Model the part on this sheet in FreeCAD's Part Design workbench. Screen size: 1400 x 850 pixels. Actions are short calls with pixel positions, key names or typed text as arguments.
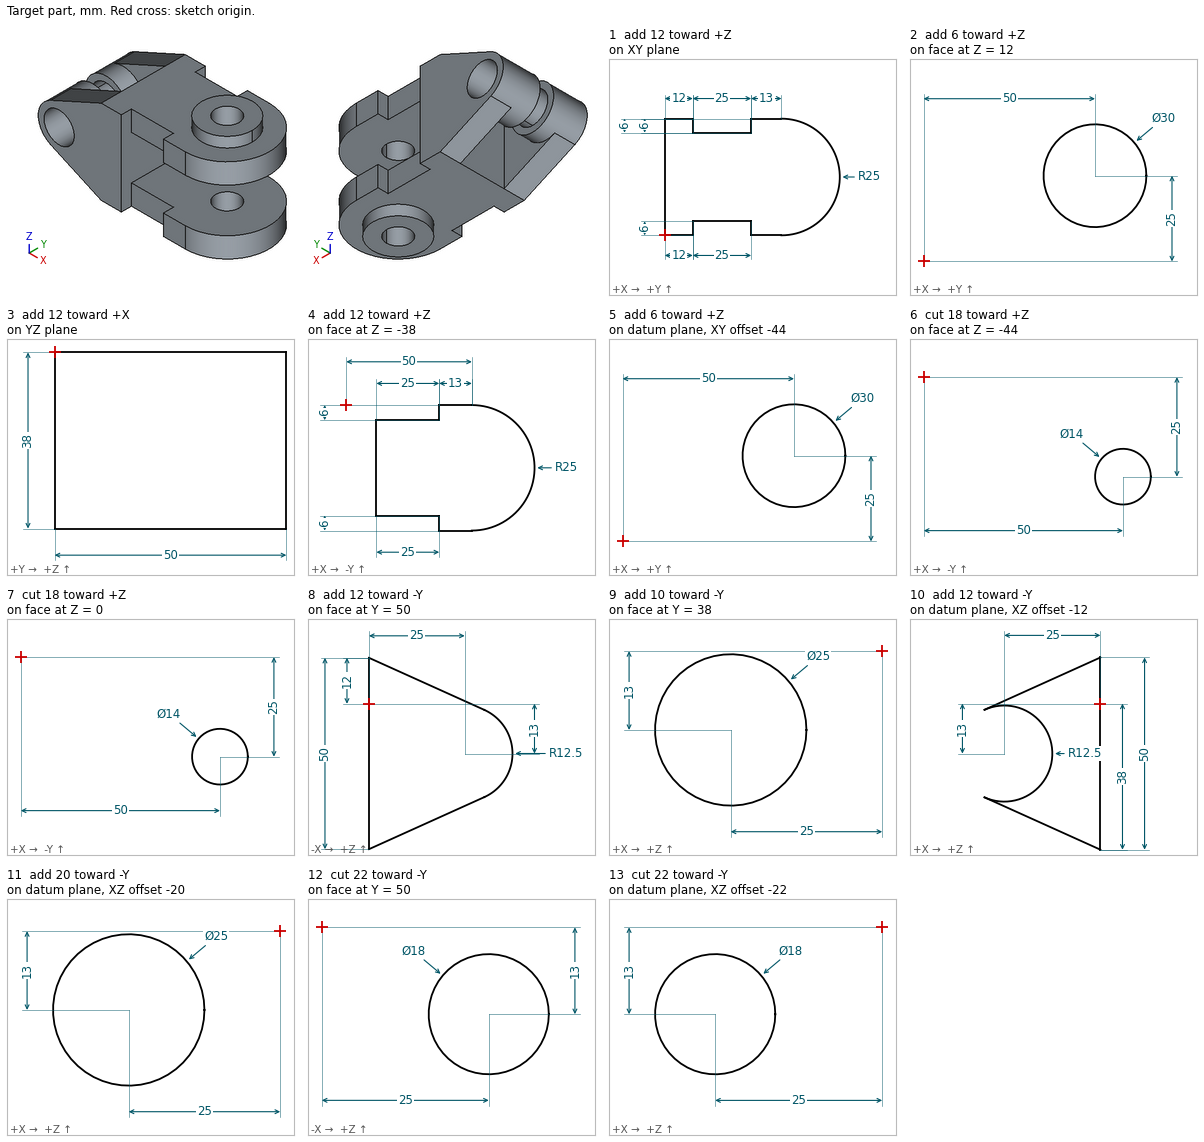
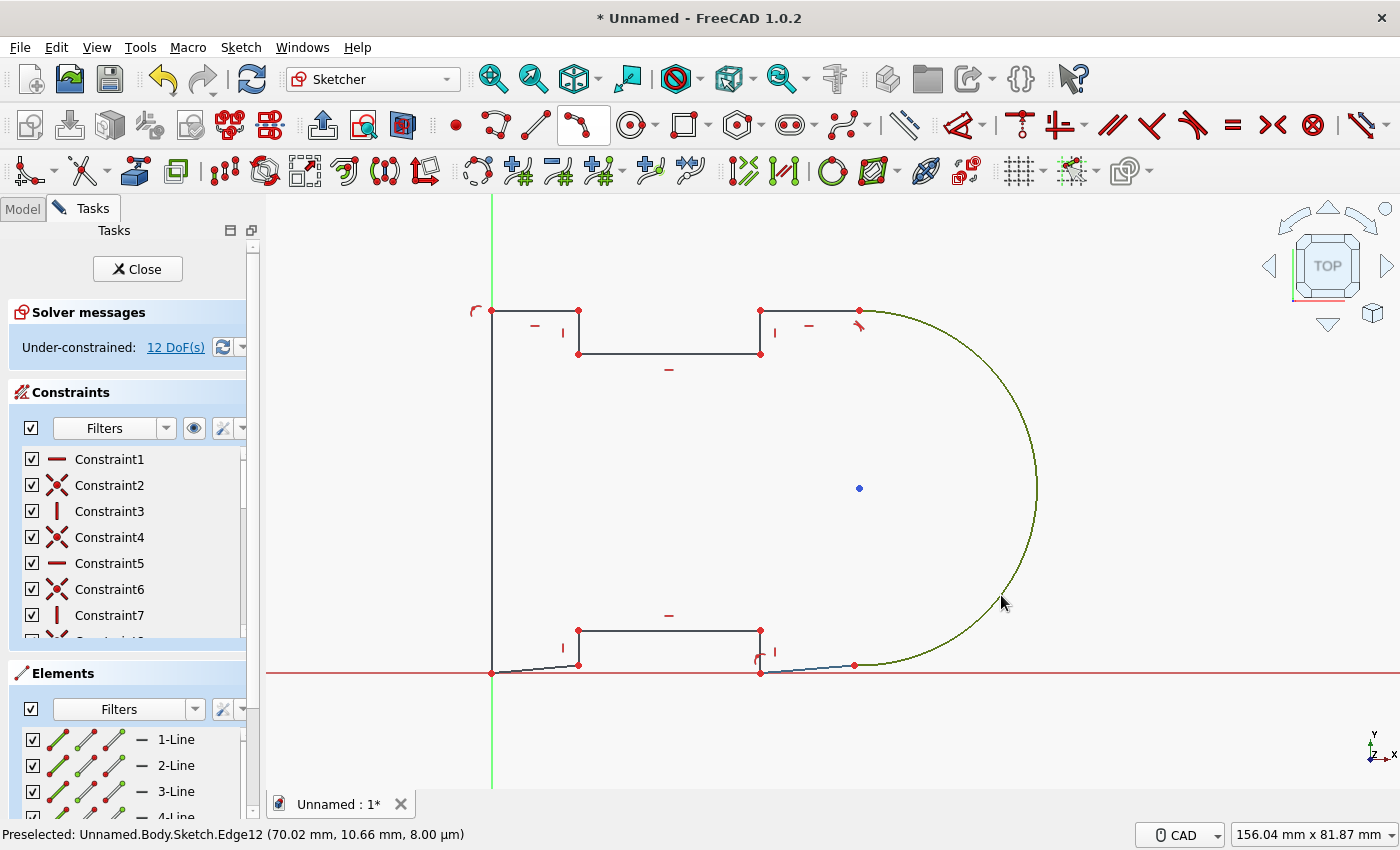
click(1194, 126)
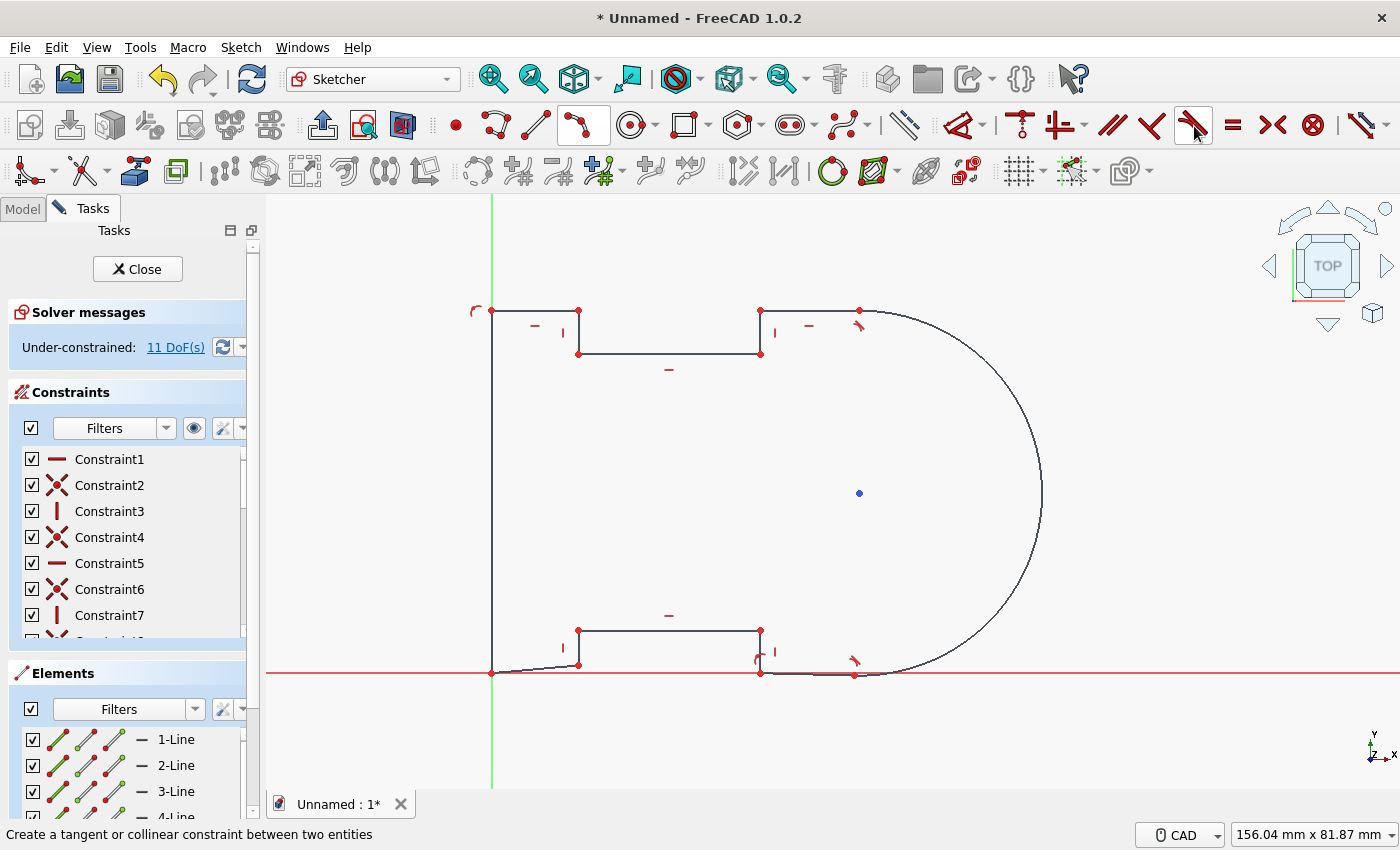
click(518, 671)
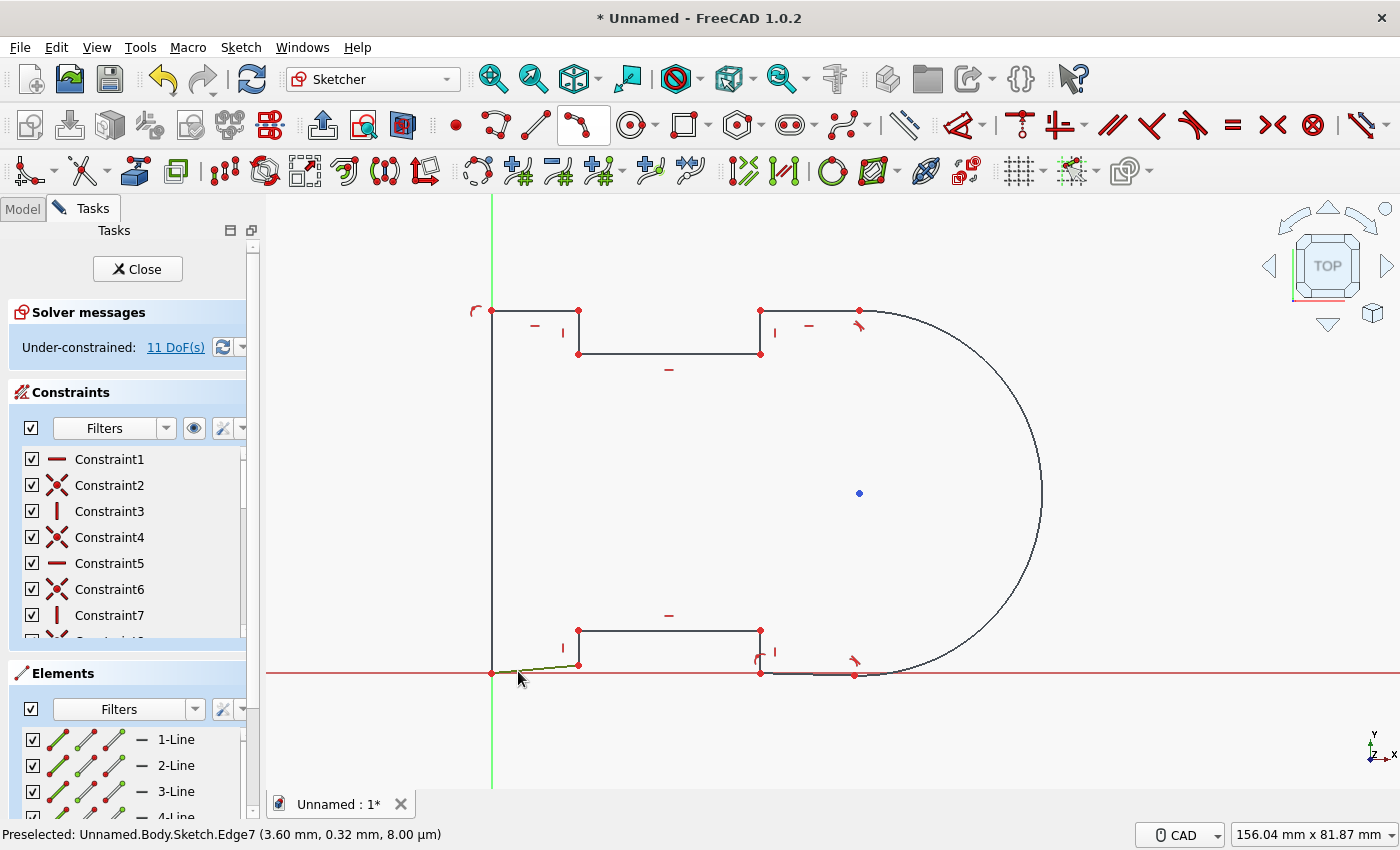
key(h)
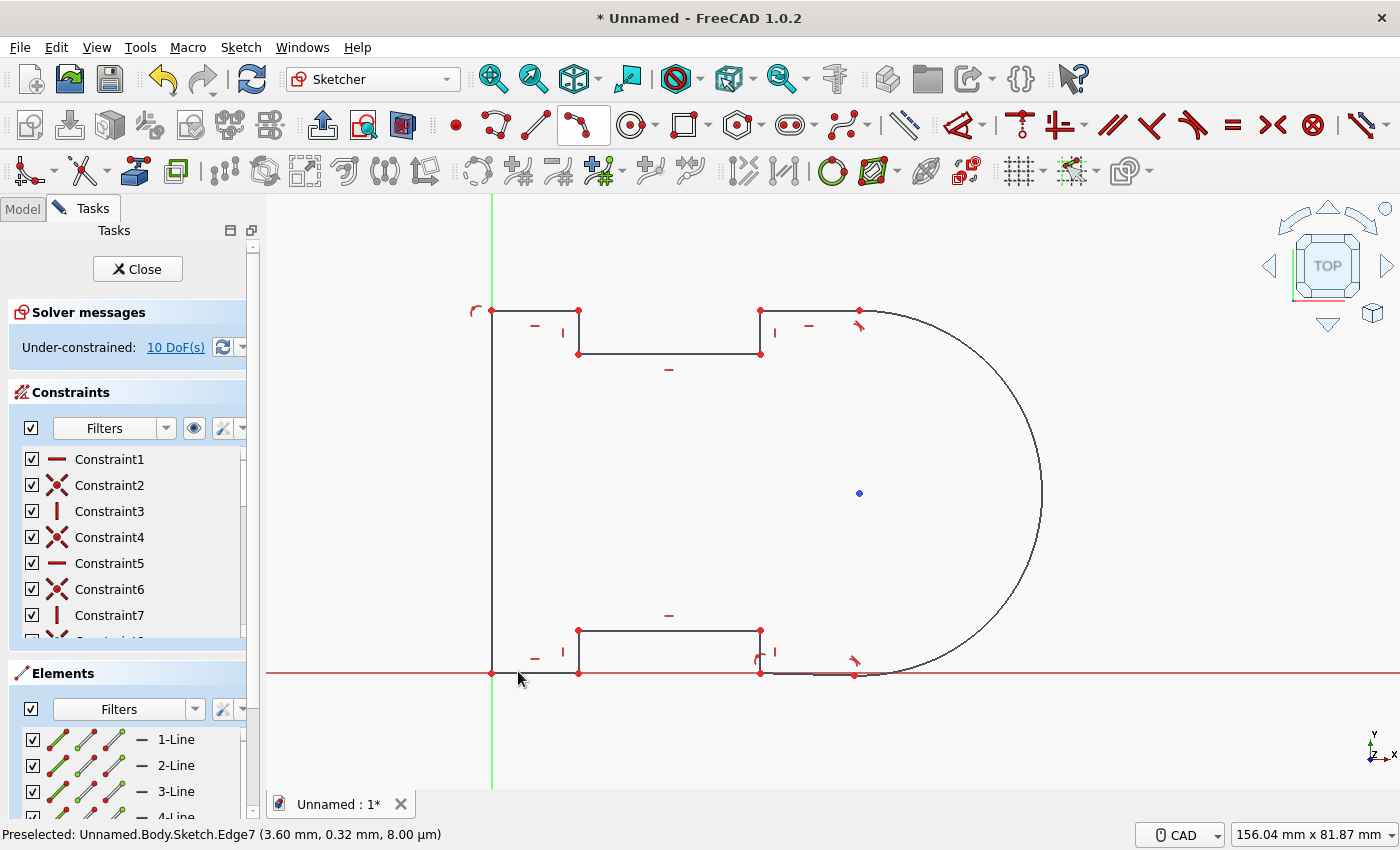
click(789, 674)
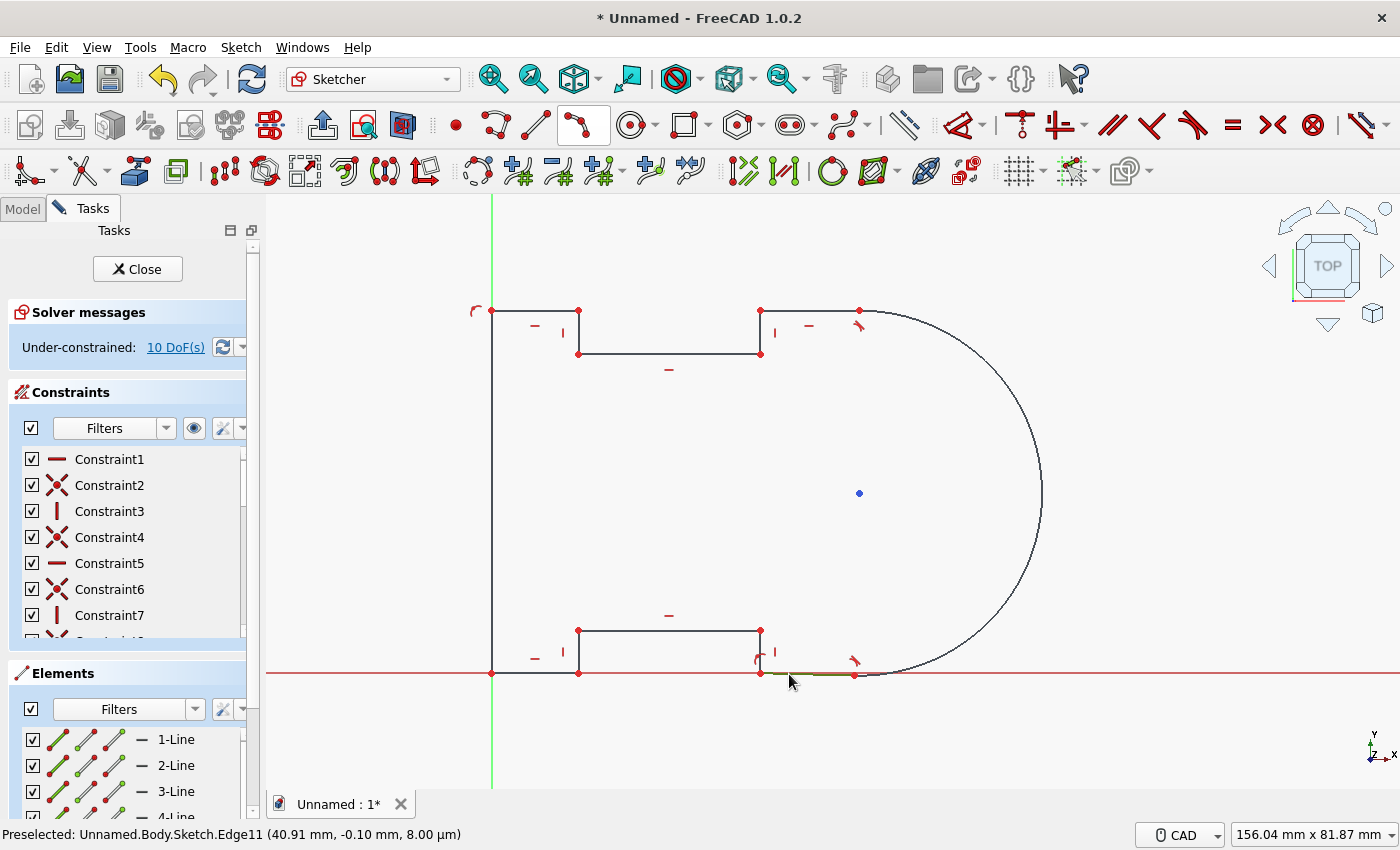
click(1086, 126)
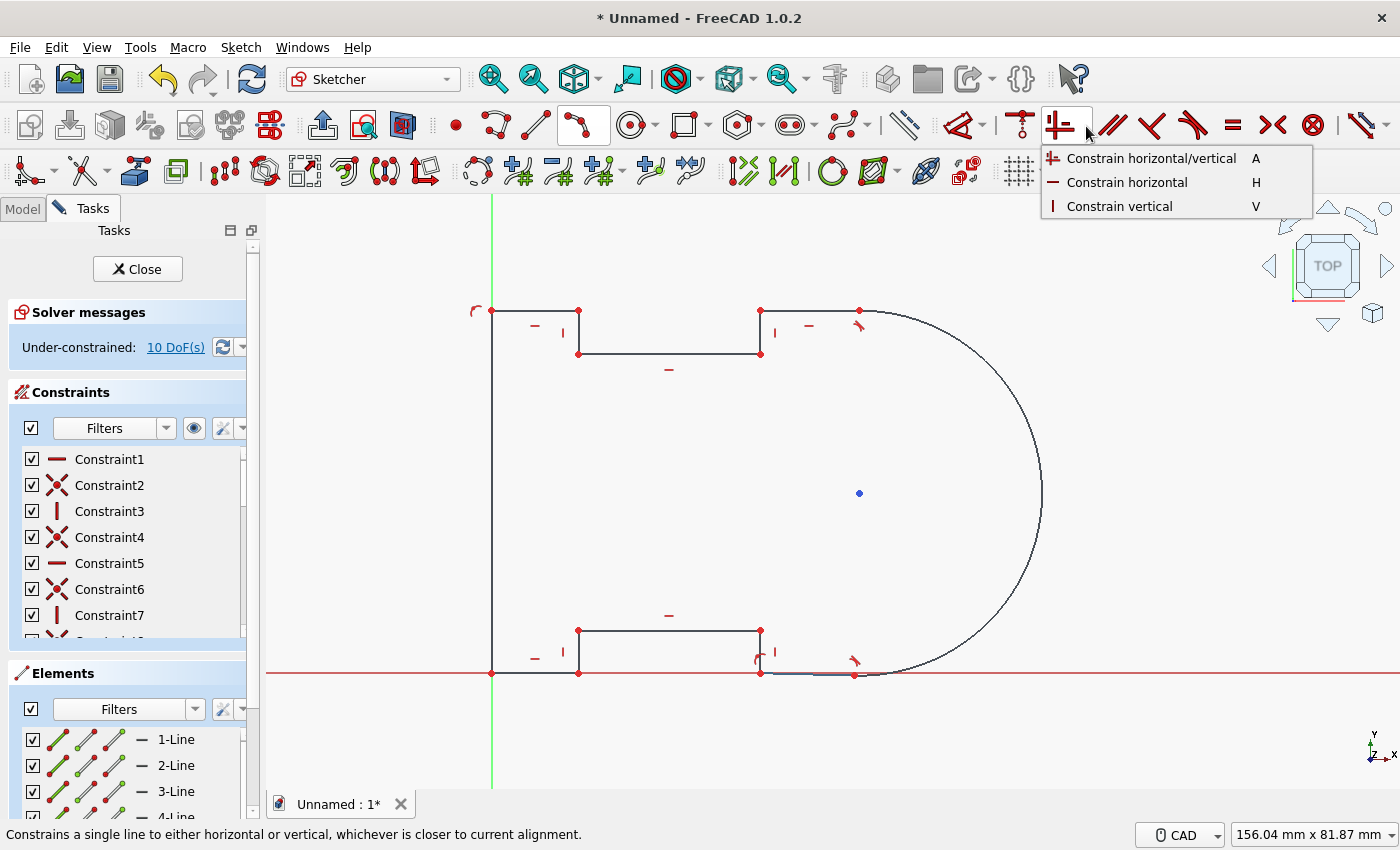
click(1177, 182)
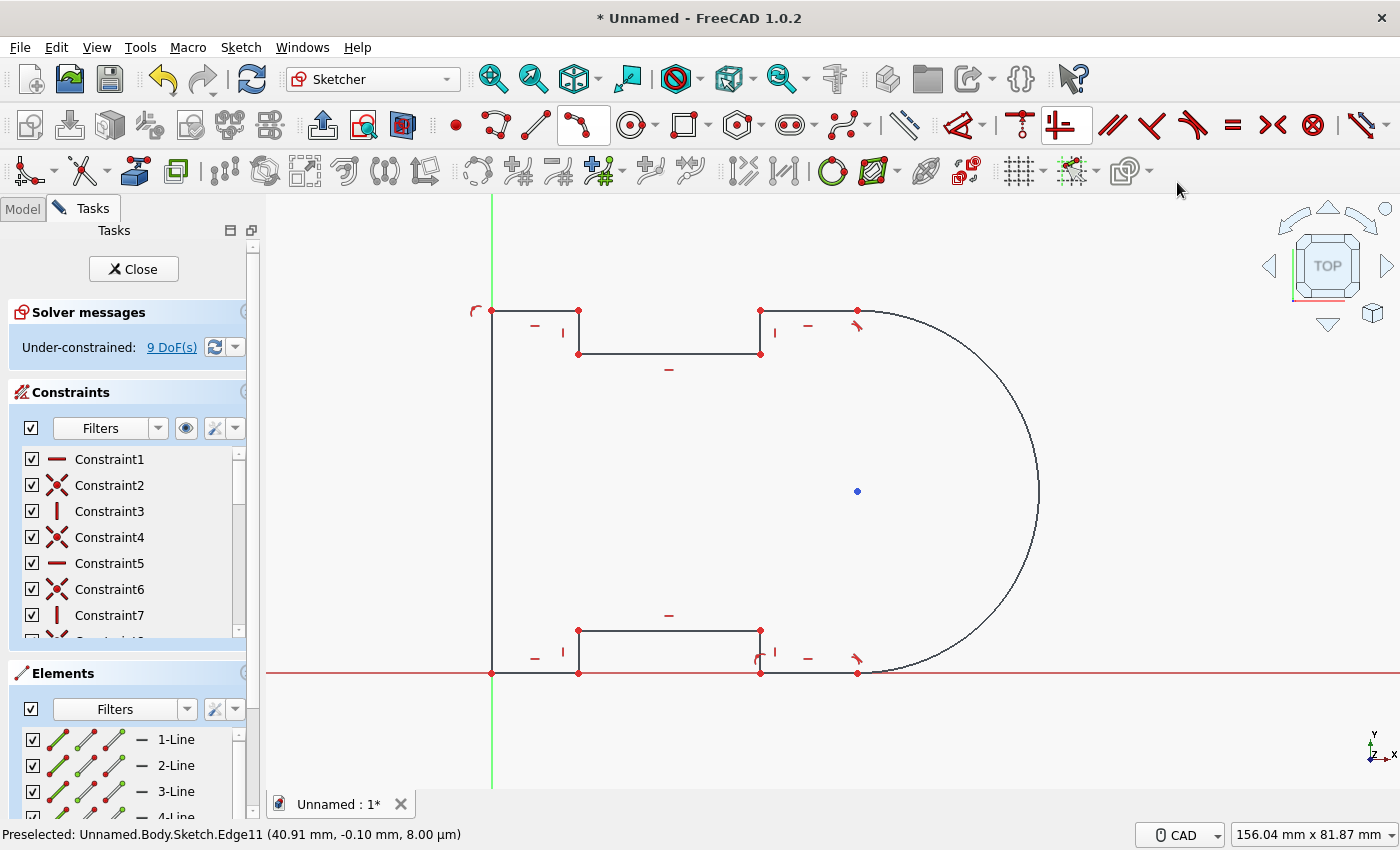
click(958, 126)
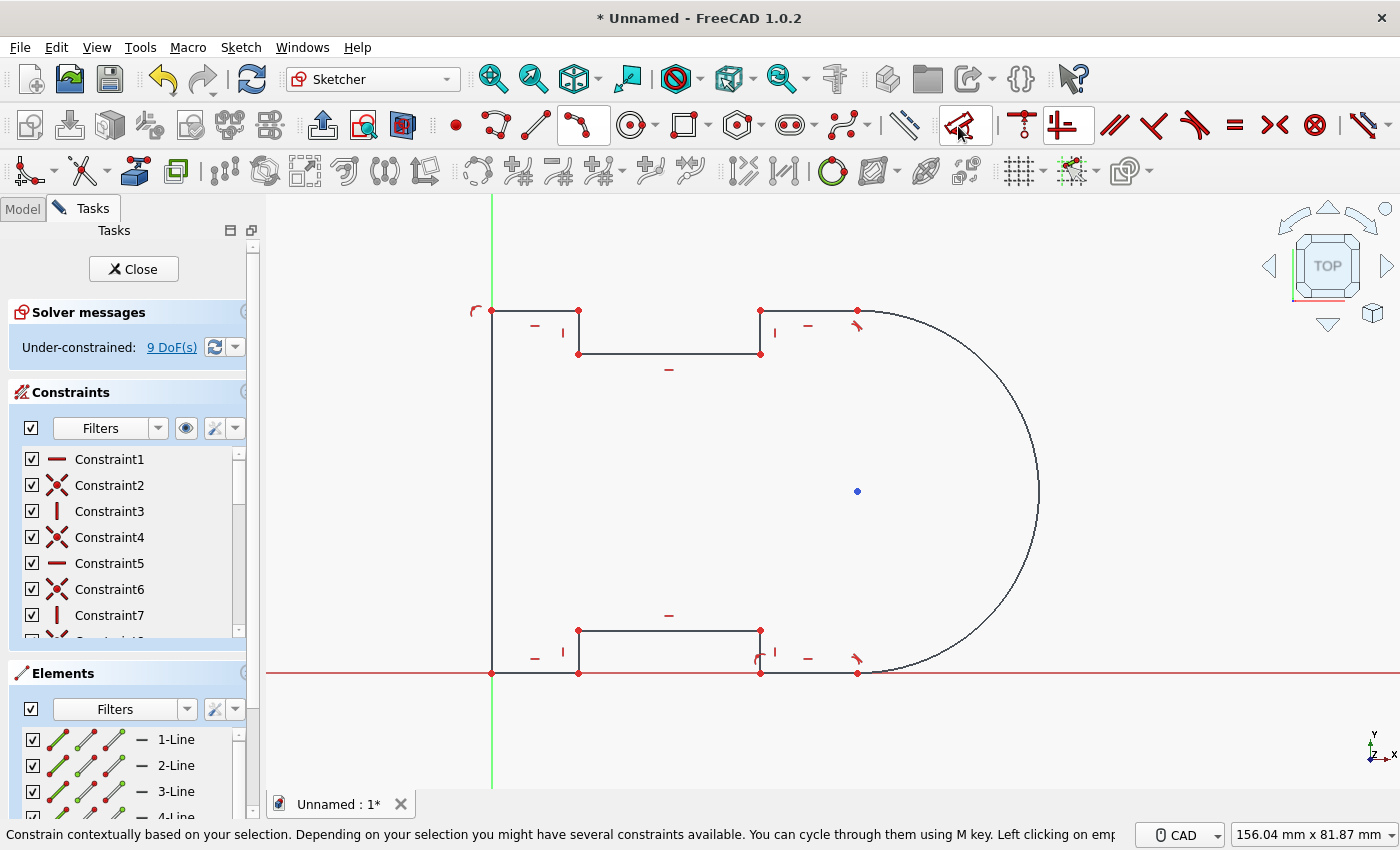
click(1004, 598)
click(1030, 617)